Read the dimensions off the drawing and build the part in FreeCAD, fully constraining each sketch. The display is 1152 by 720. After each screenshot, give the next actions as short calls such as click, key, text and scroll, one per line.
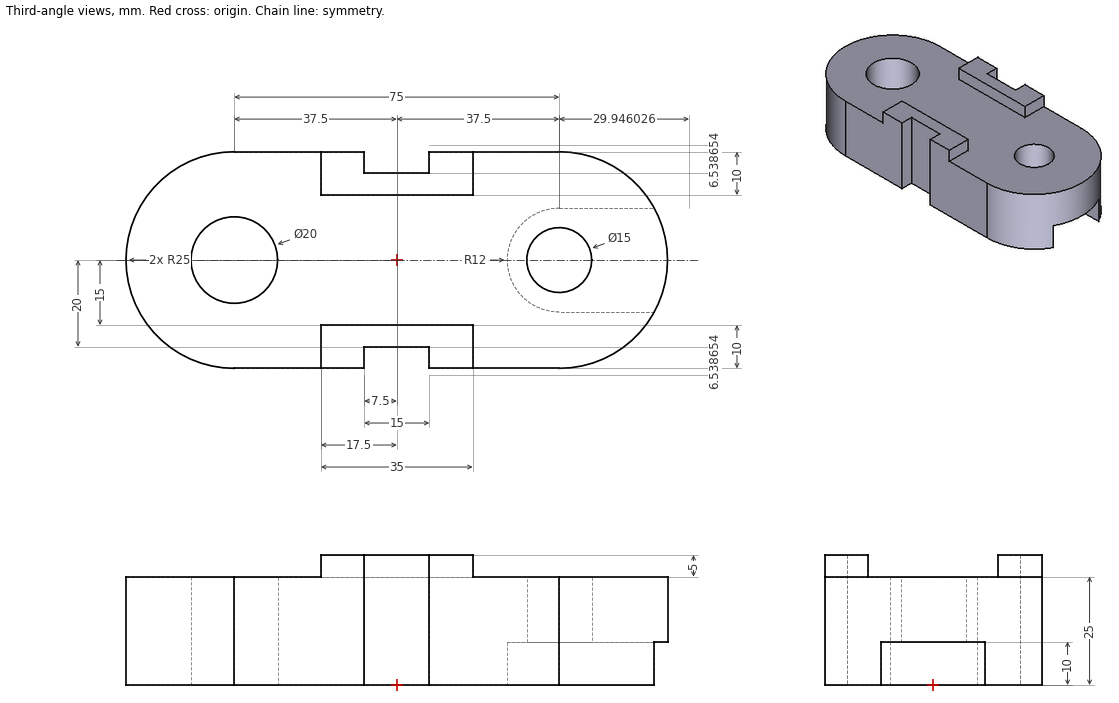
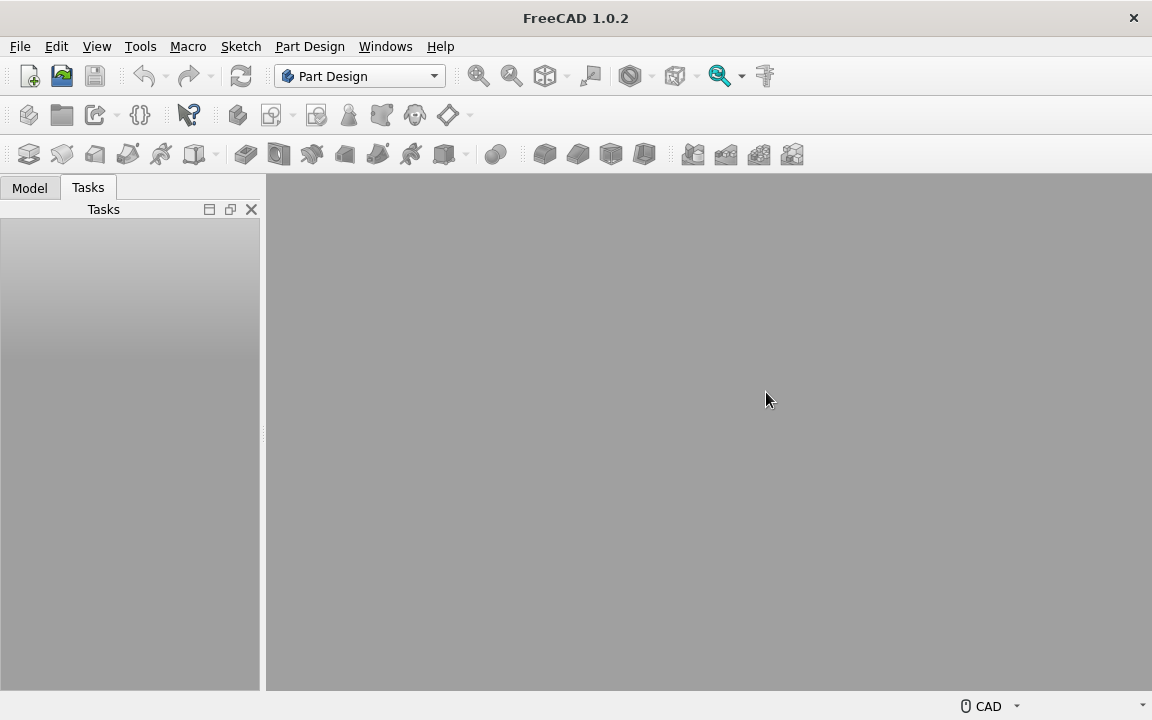
click(29, 76)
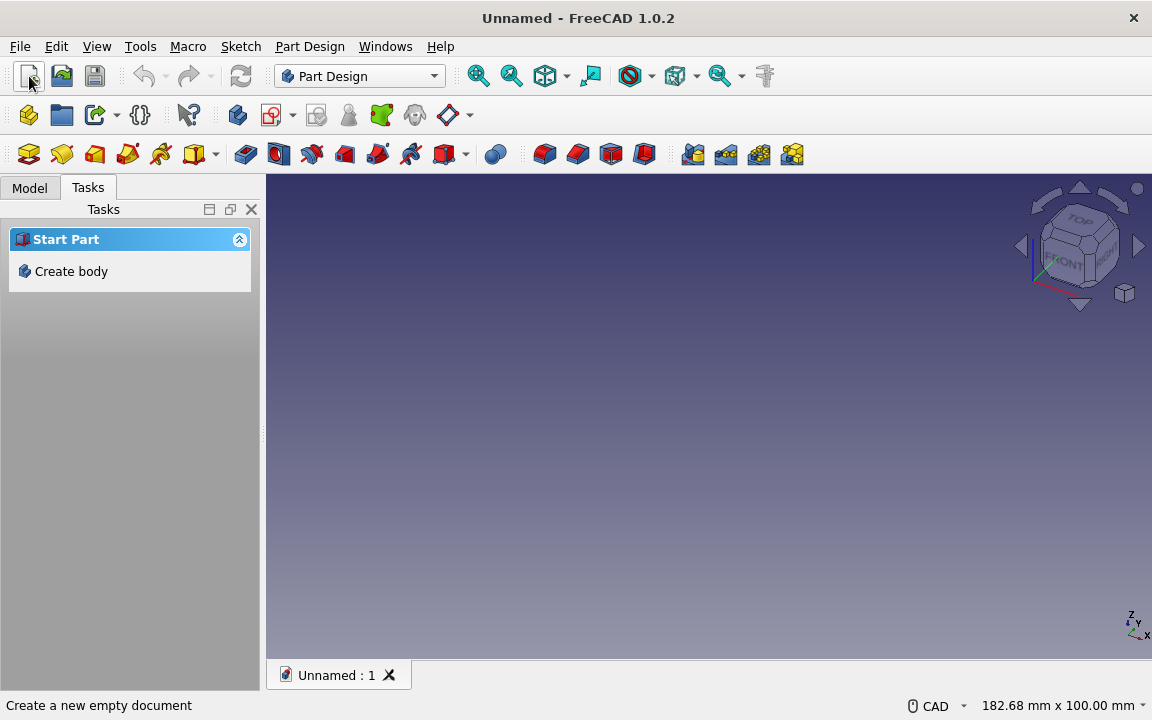
click(270, 116)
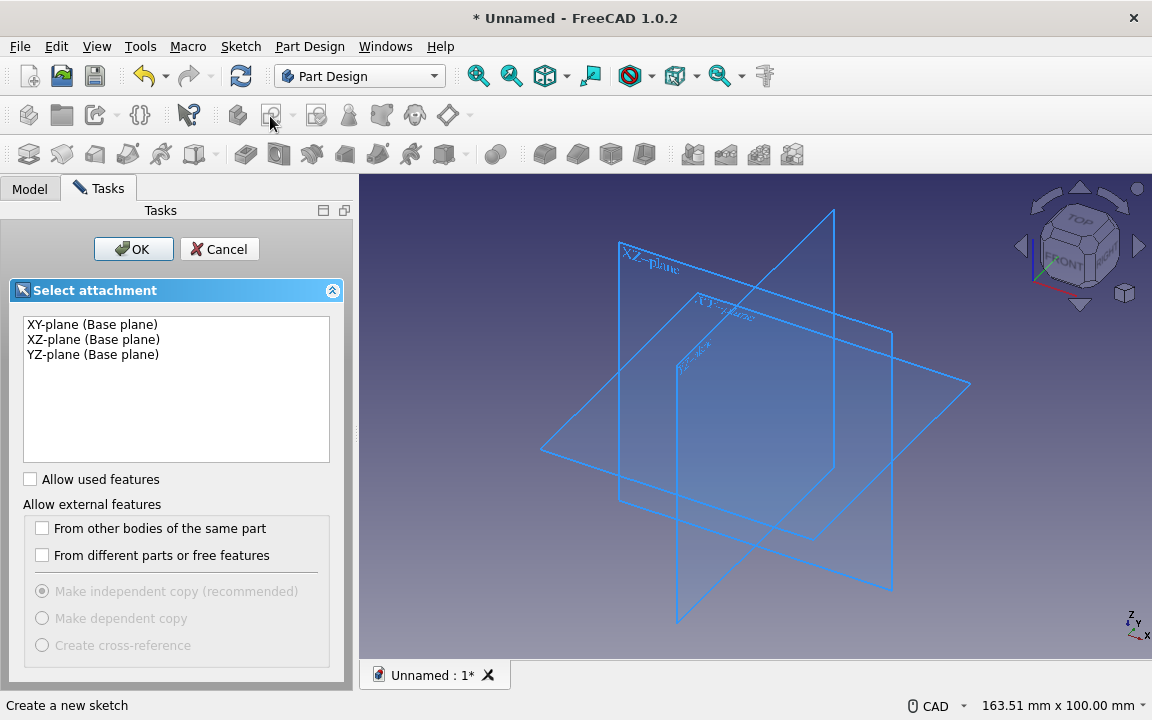
click(84, 324)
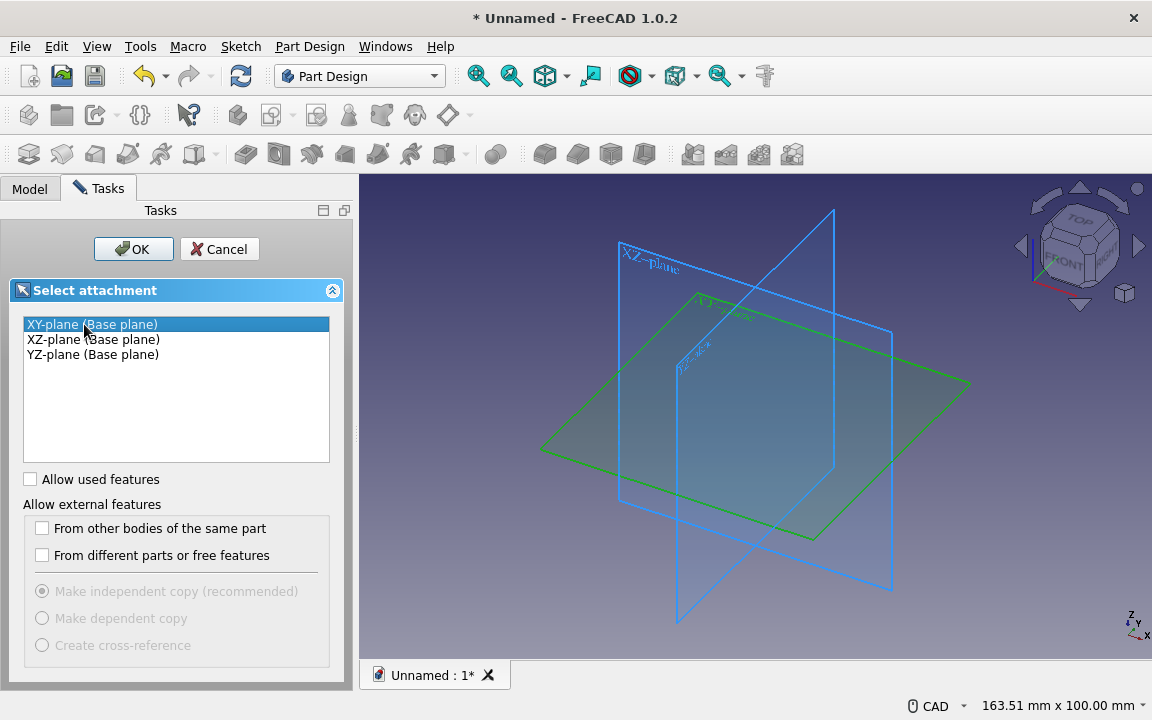
click(134, 249)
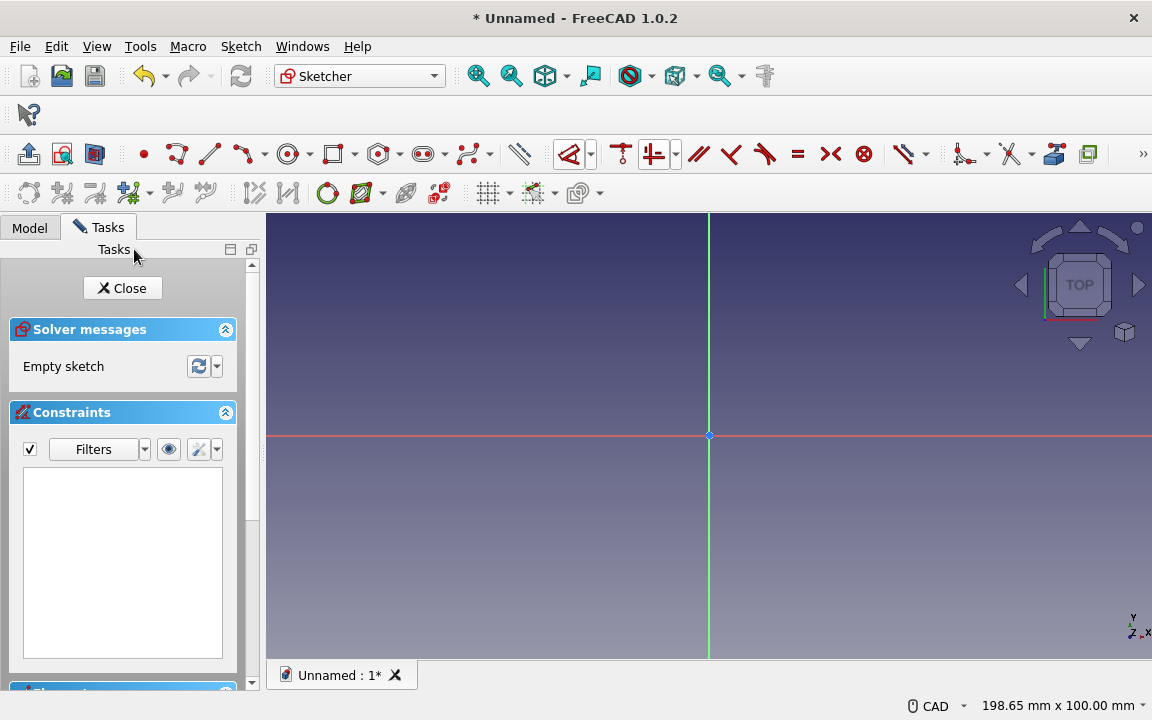
scroll(331, 436, down, 1)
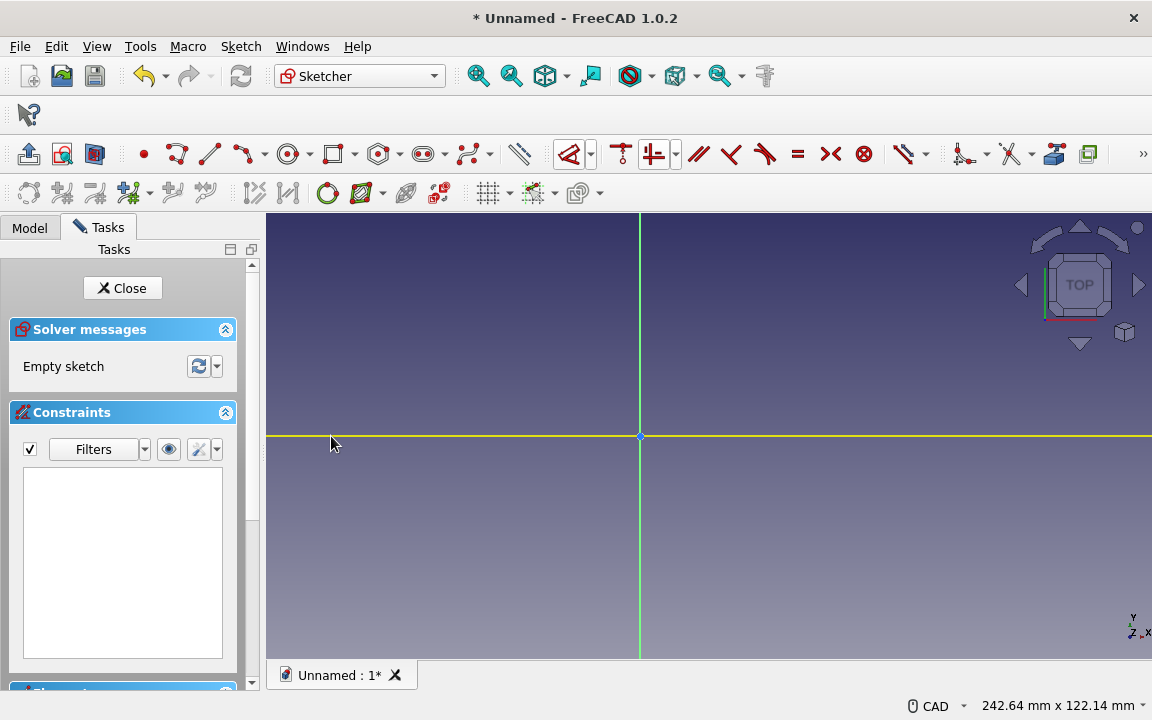
click(422, 154)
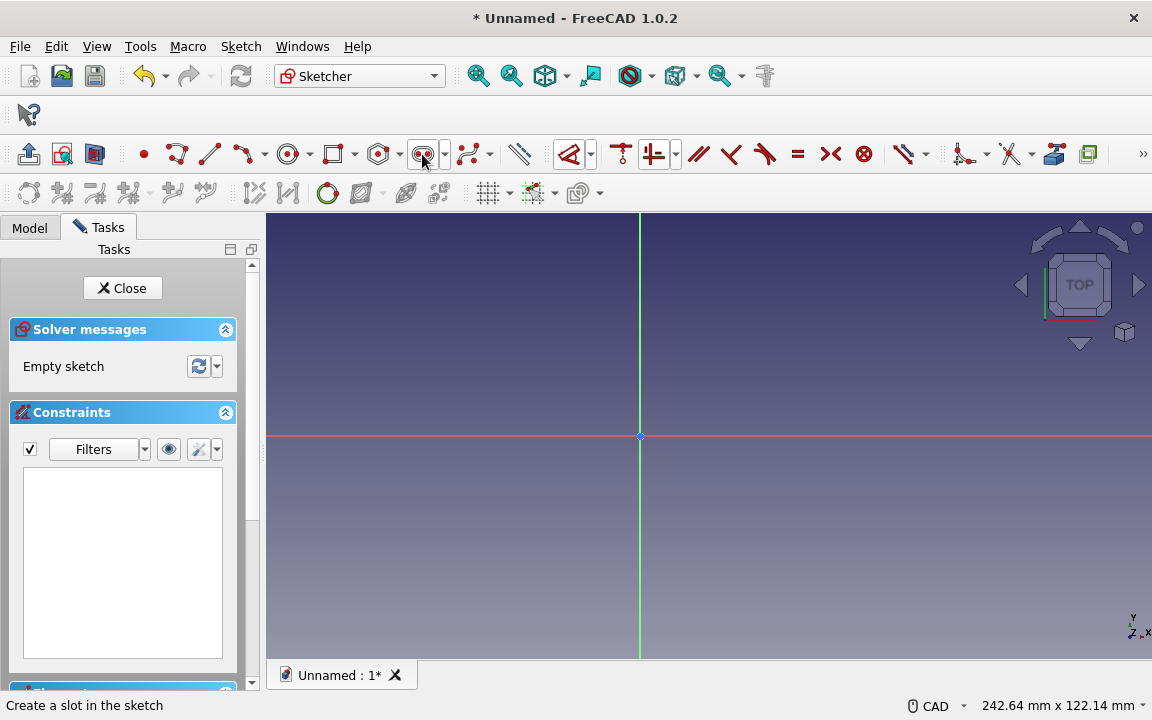
click(504, 436)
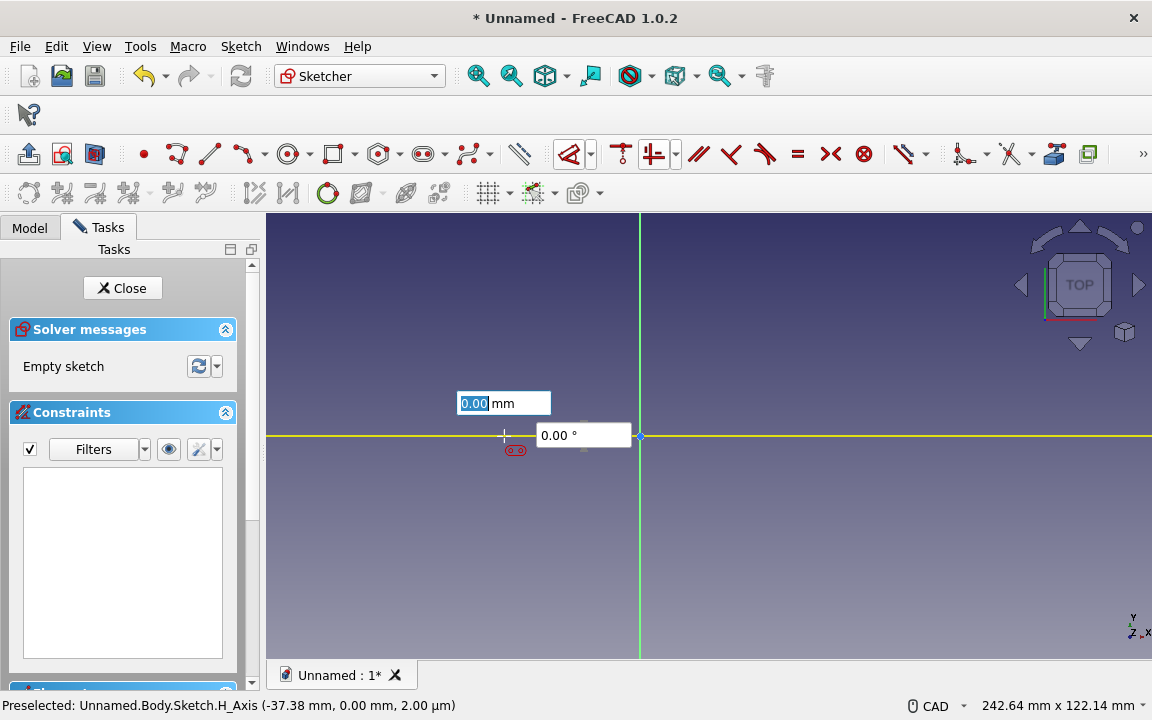
click(777, 427)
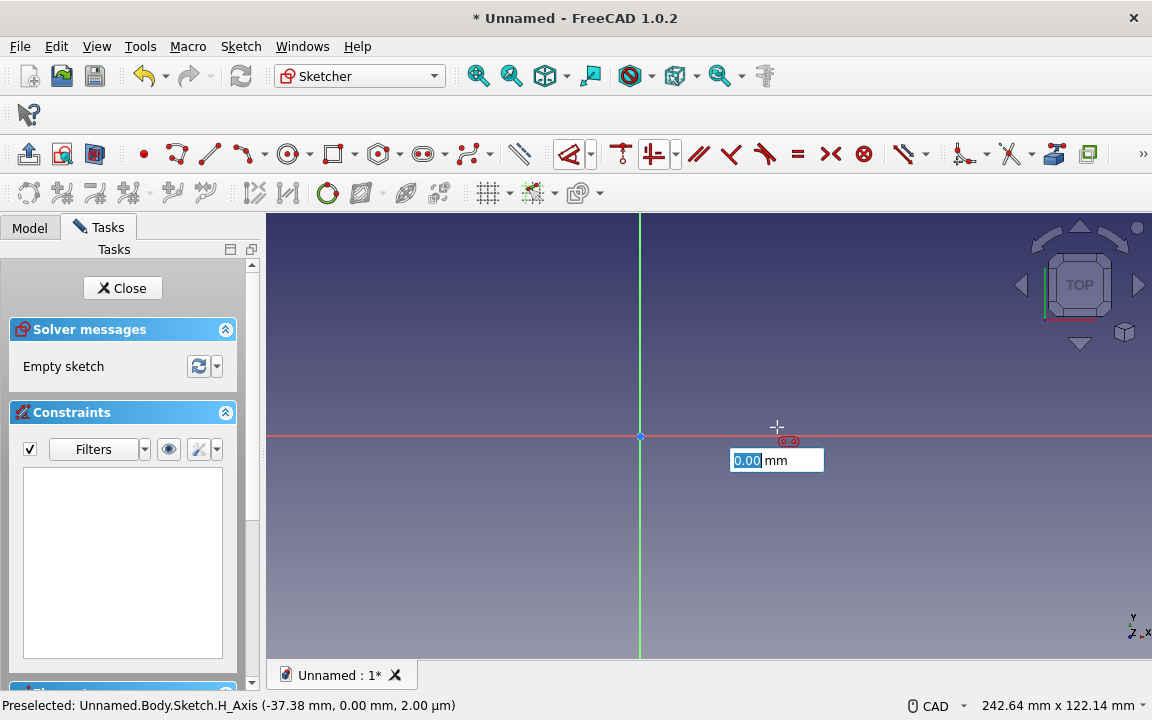
click(682, 345)
key(Escape)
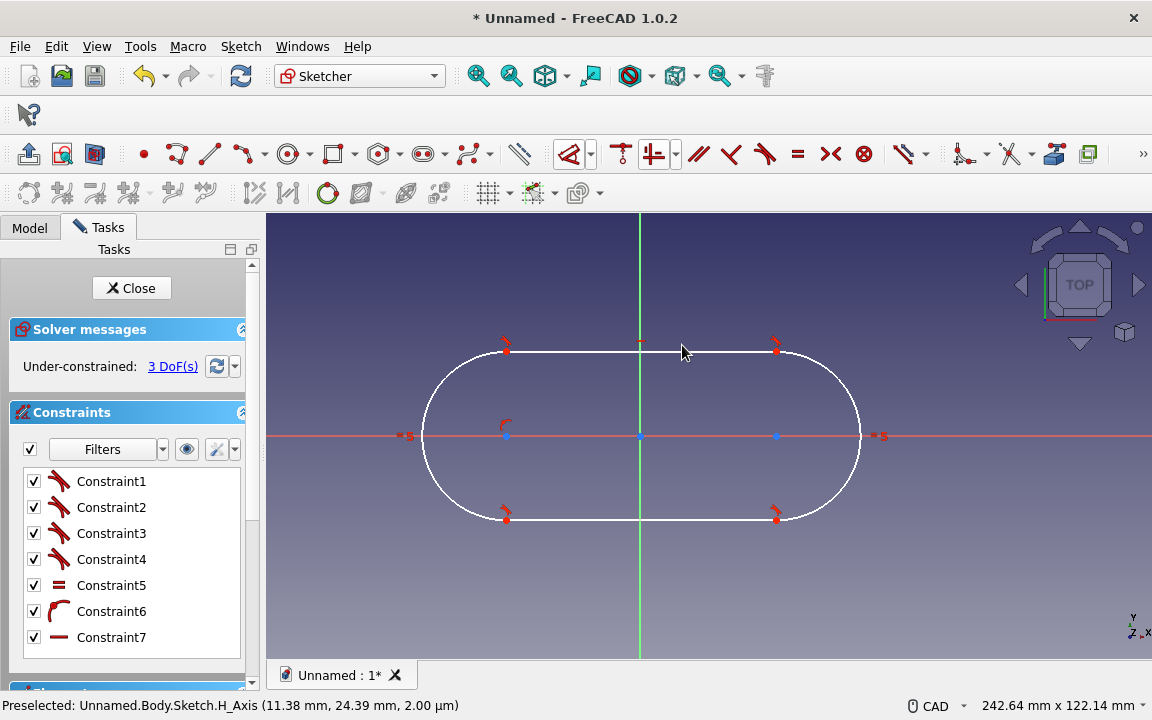
click(568, 154)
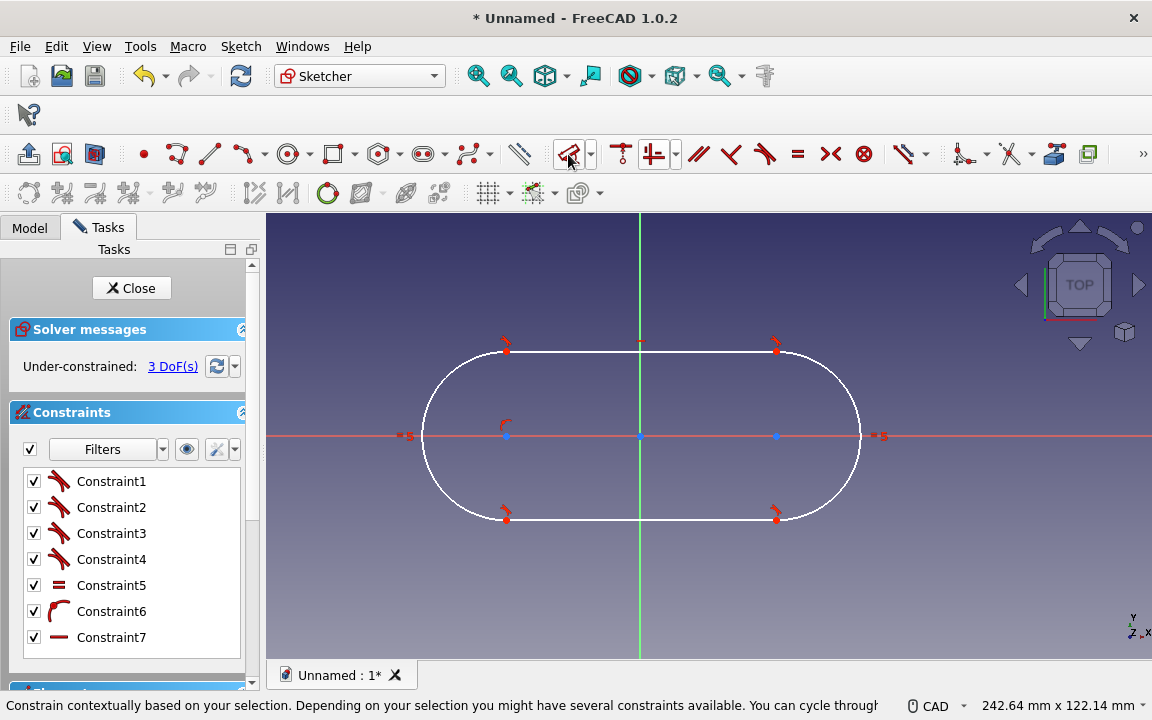
click(438, 387)
click(412, 368)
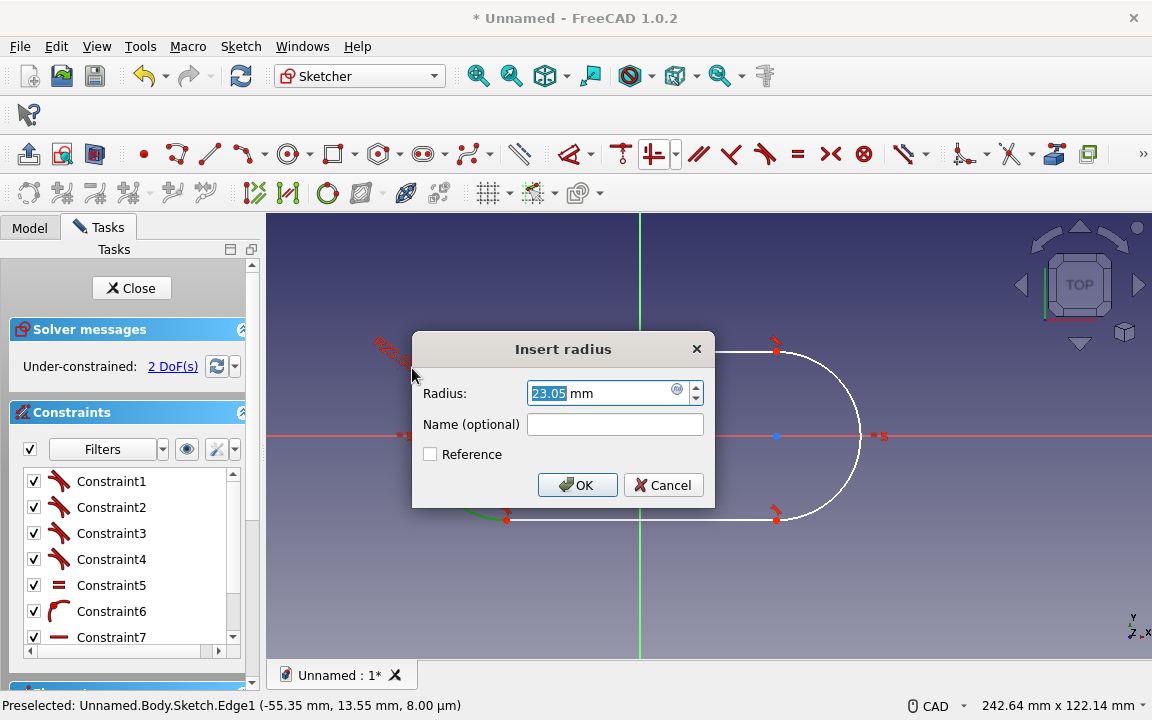
text(25)
key(Return)